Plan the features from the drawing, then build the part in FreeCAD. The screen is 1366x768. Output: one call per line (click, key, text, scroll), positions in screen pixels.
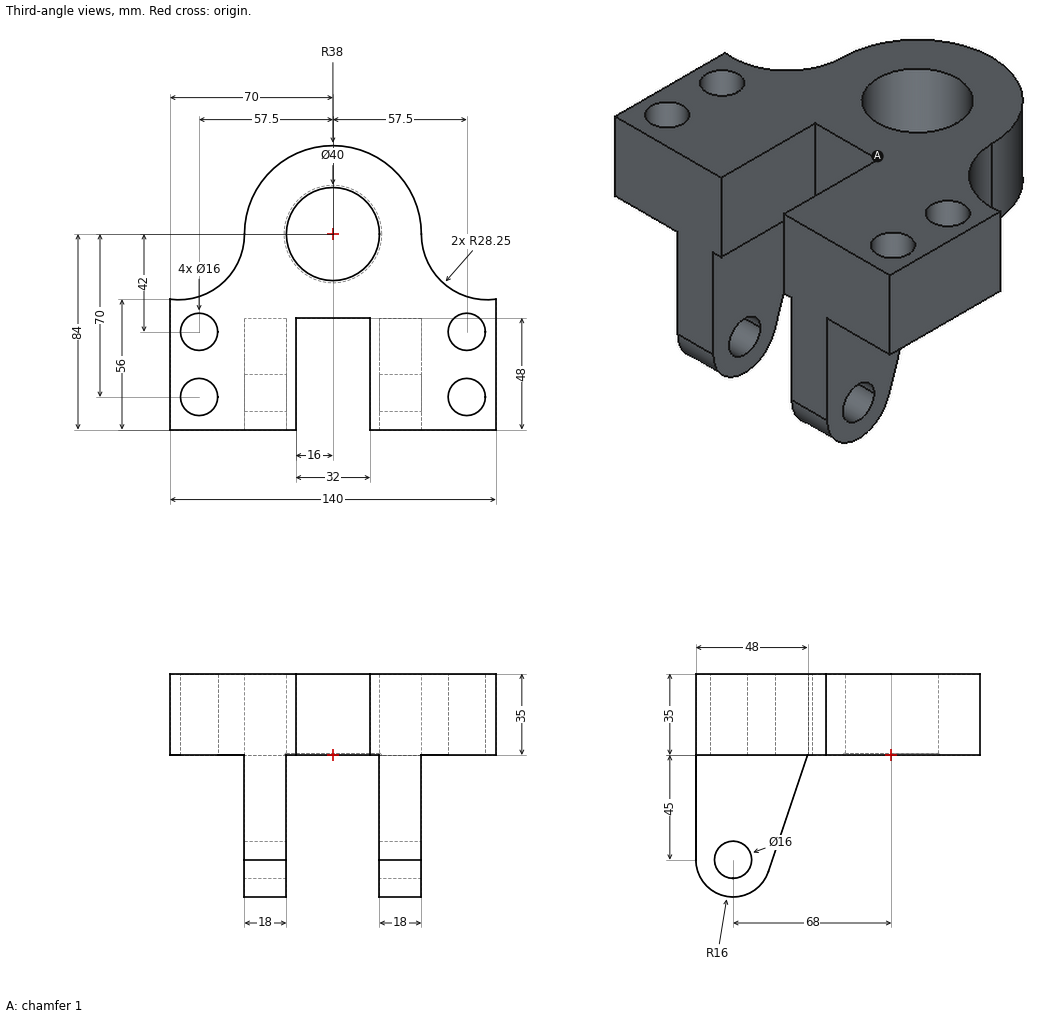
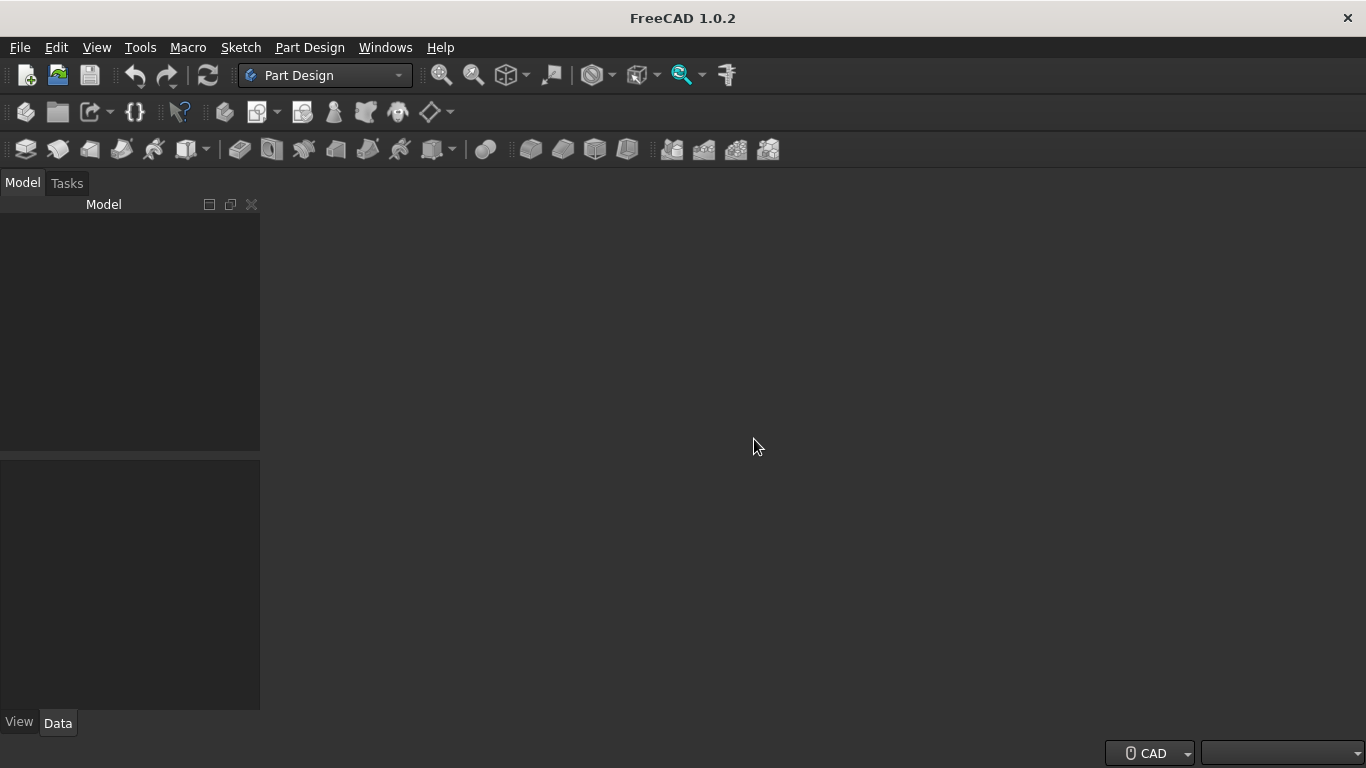
click(26, 76)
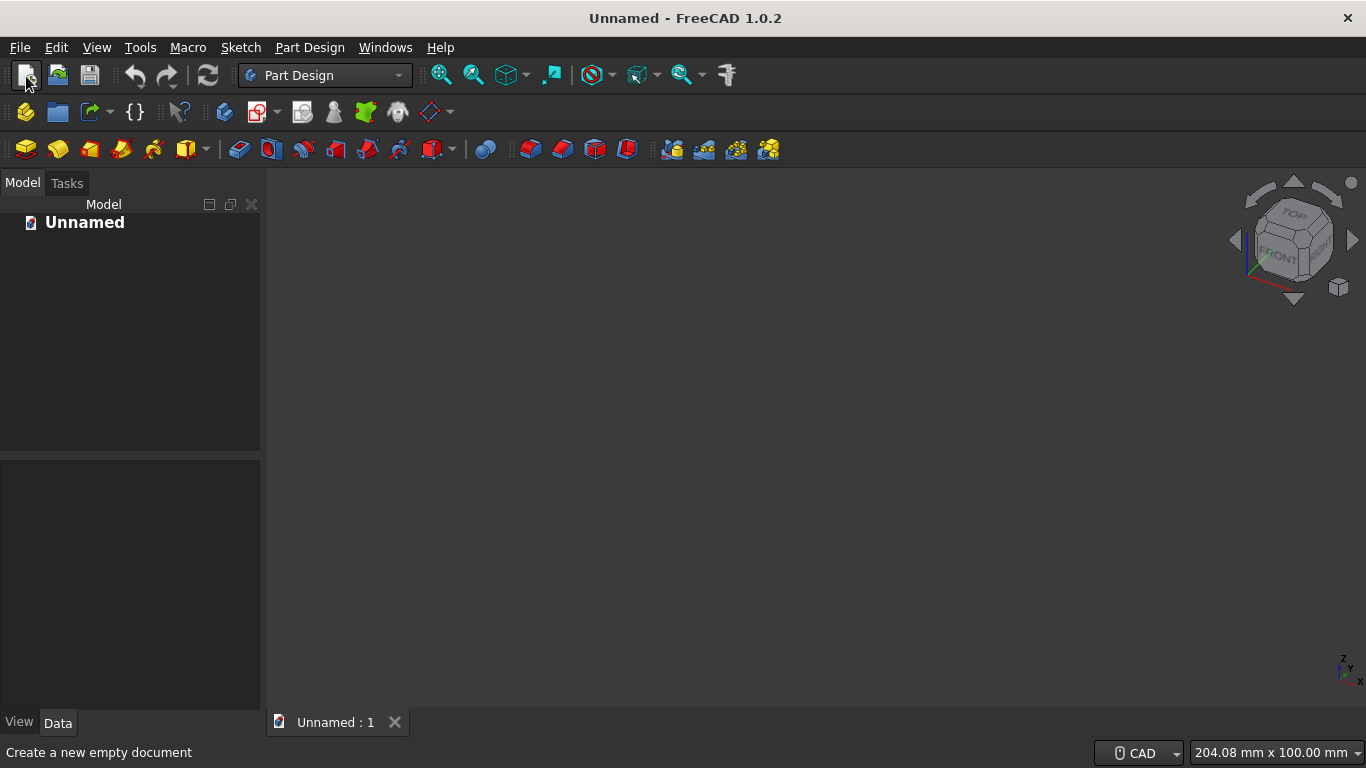
click(258, 112)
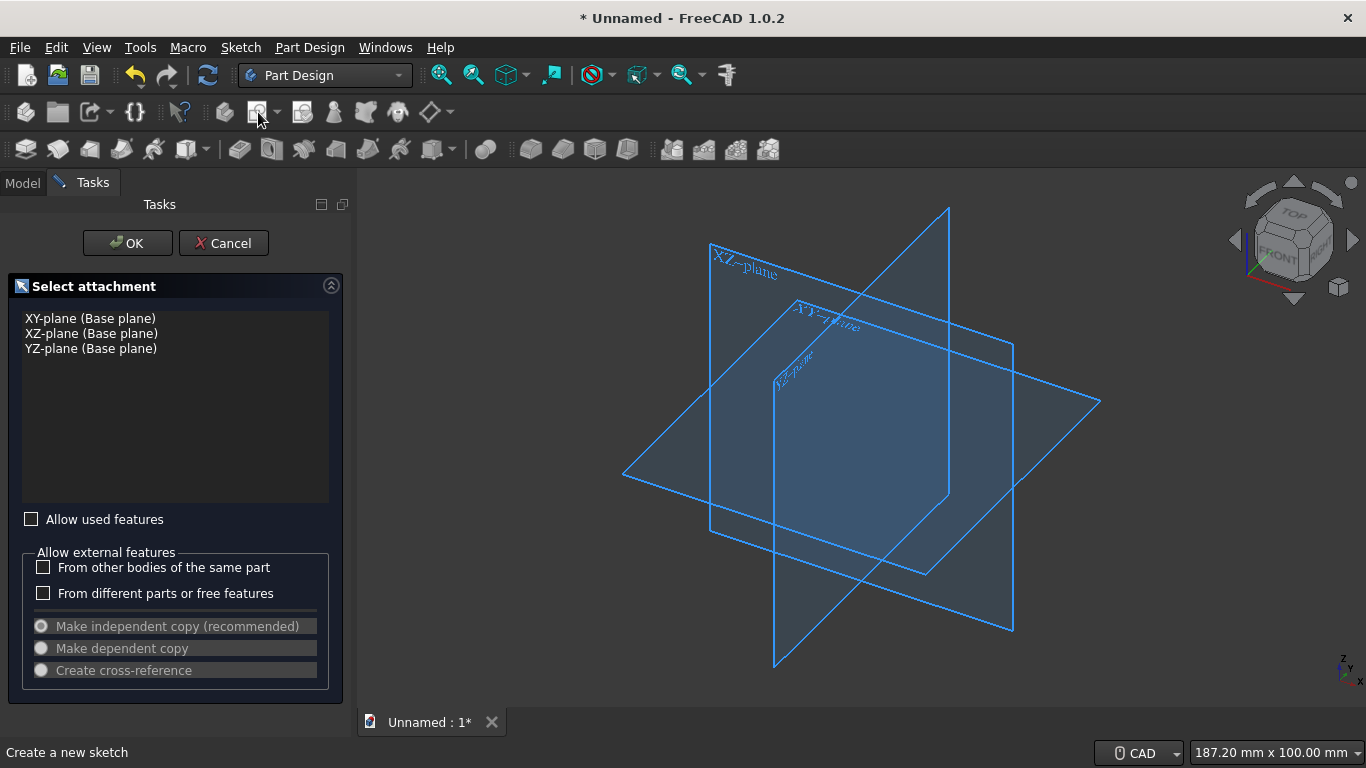
click(82, 318)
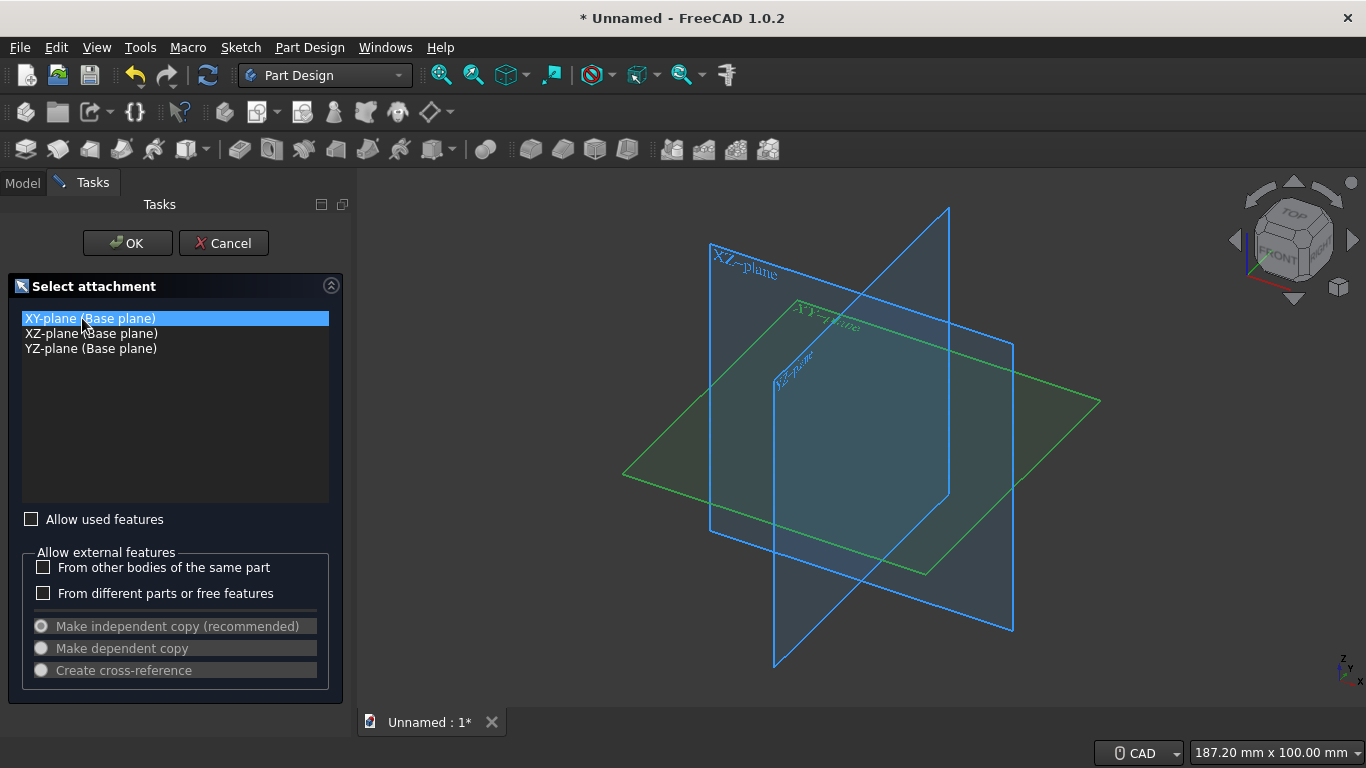
click(128, 243)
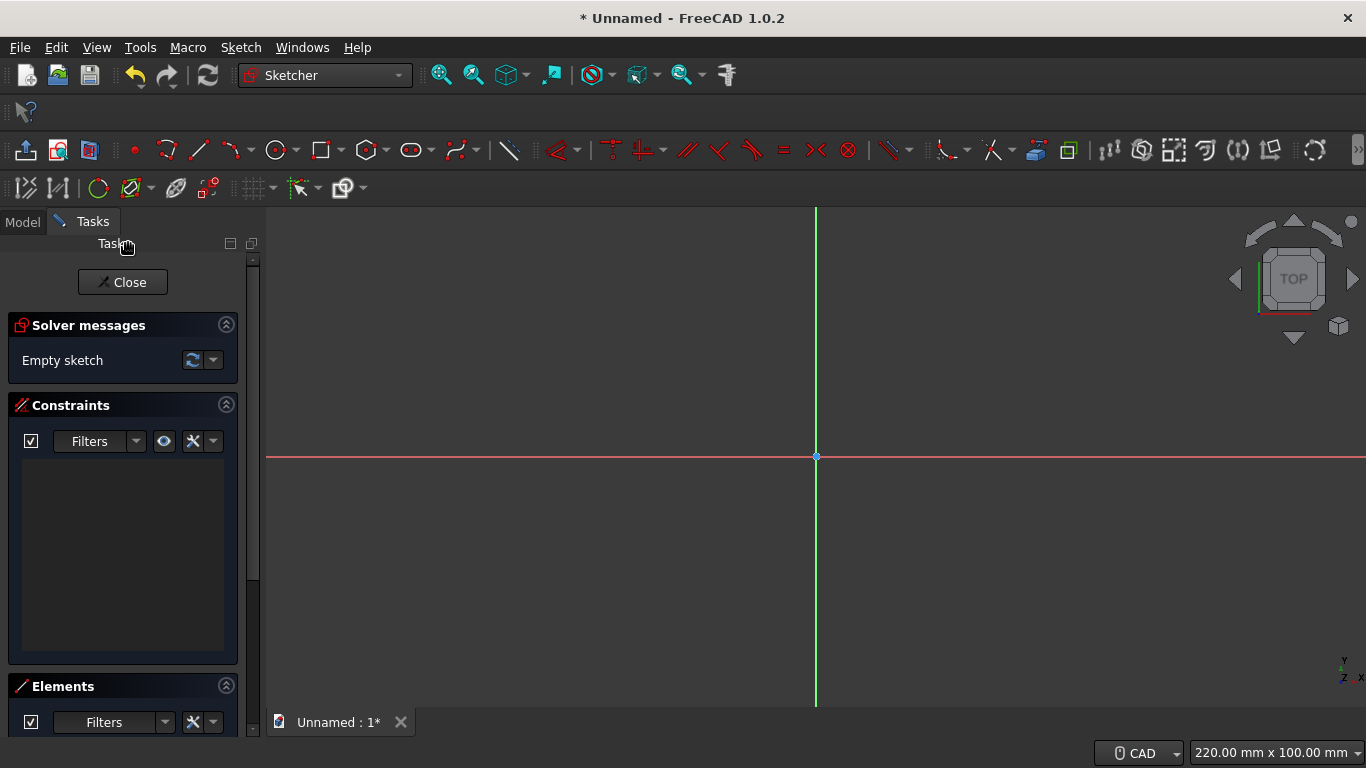
scroll(664, 317, down, 3)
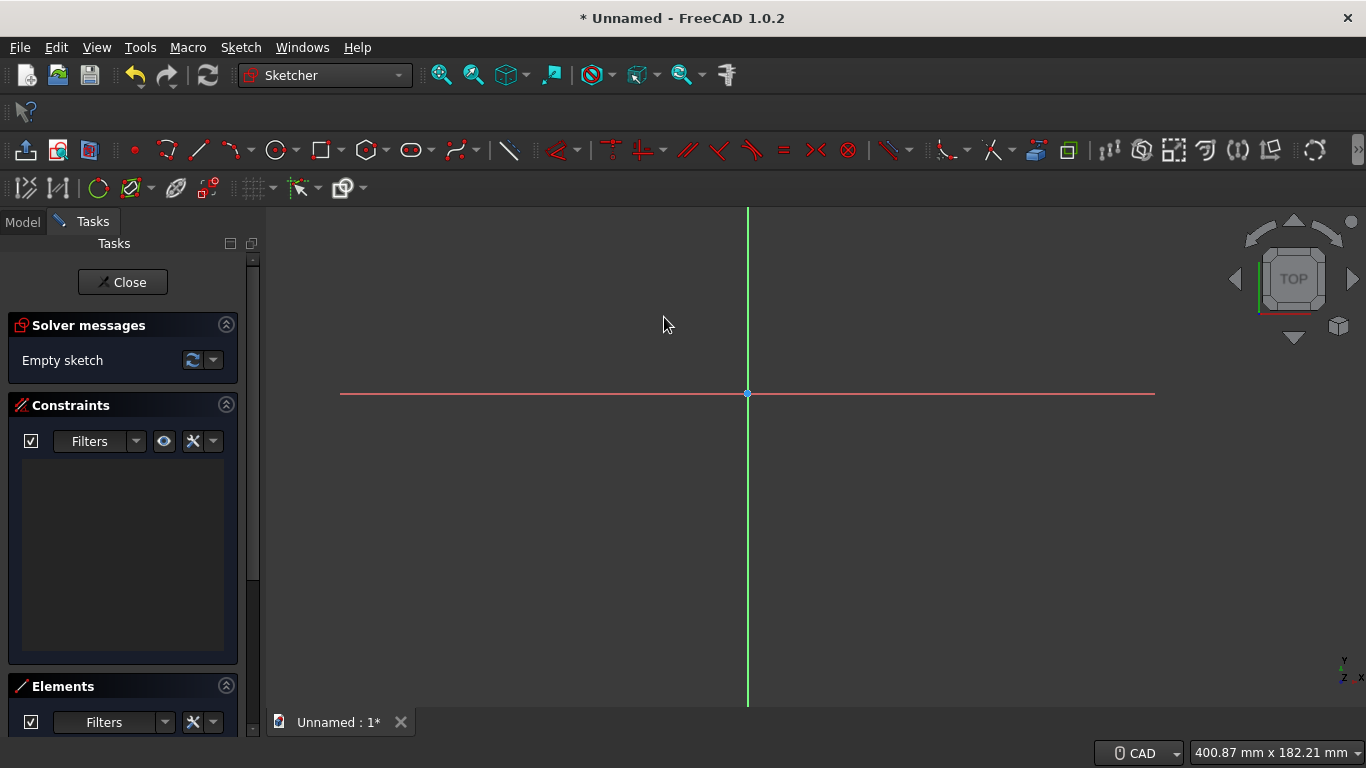
key(g)
key(m)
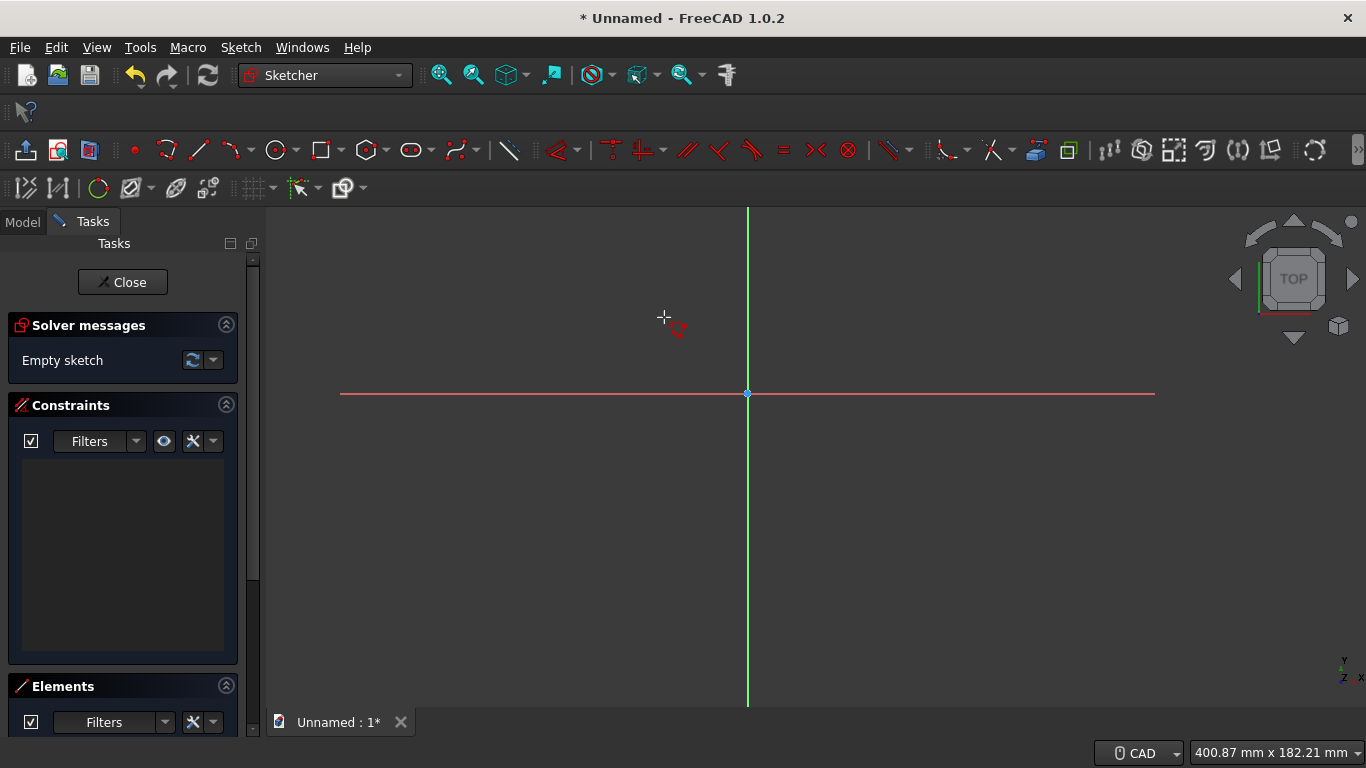
click(555, 471)
click(555, 624)
click(940, 624)
click(940, 471)
right_click(940, 471)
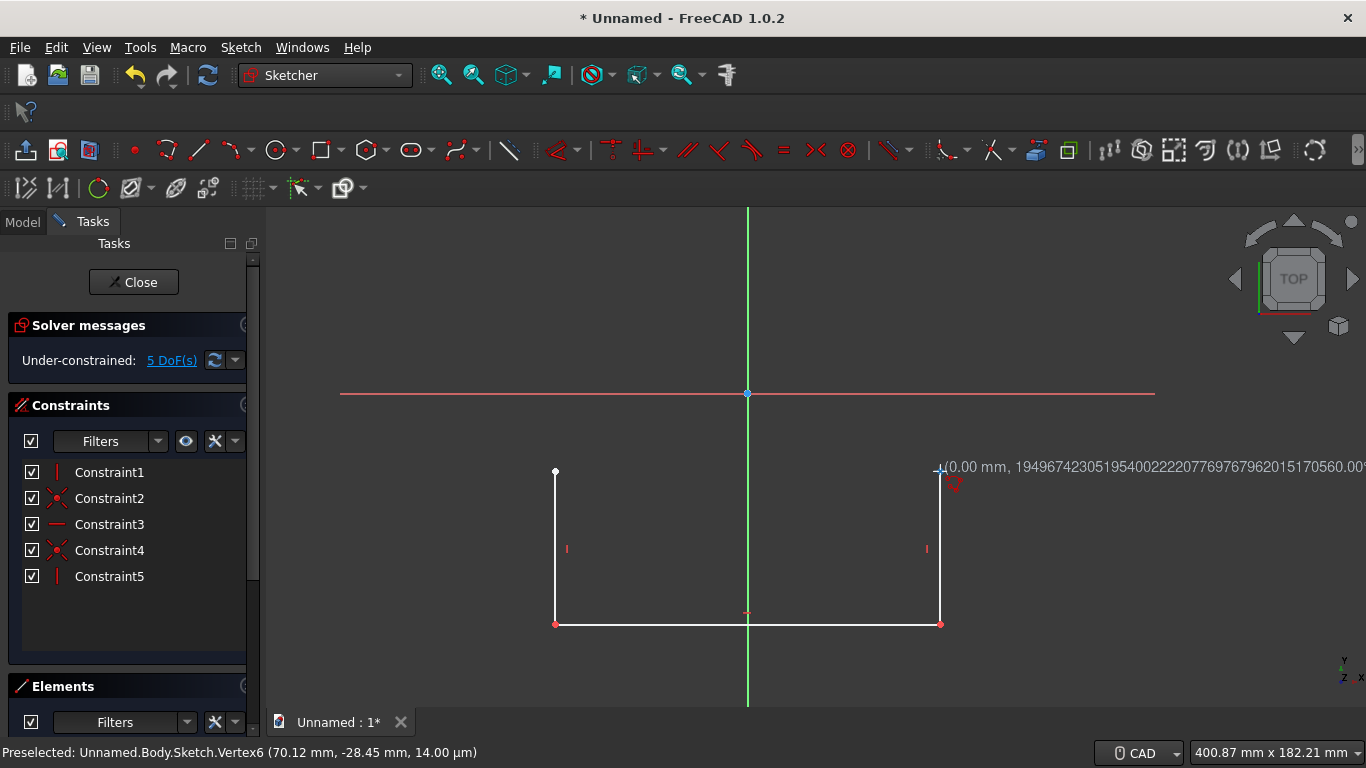
click(232, 150)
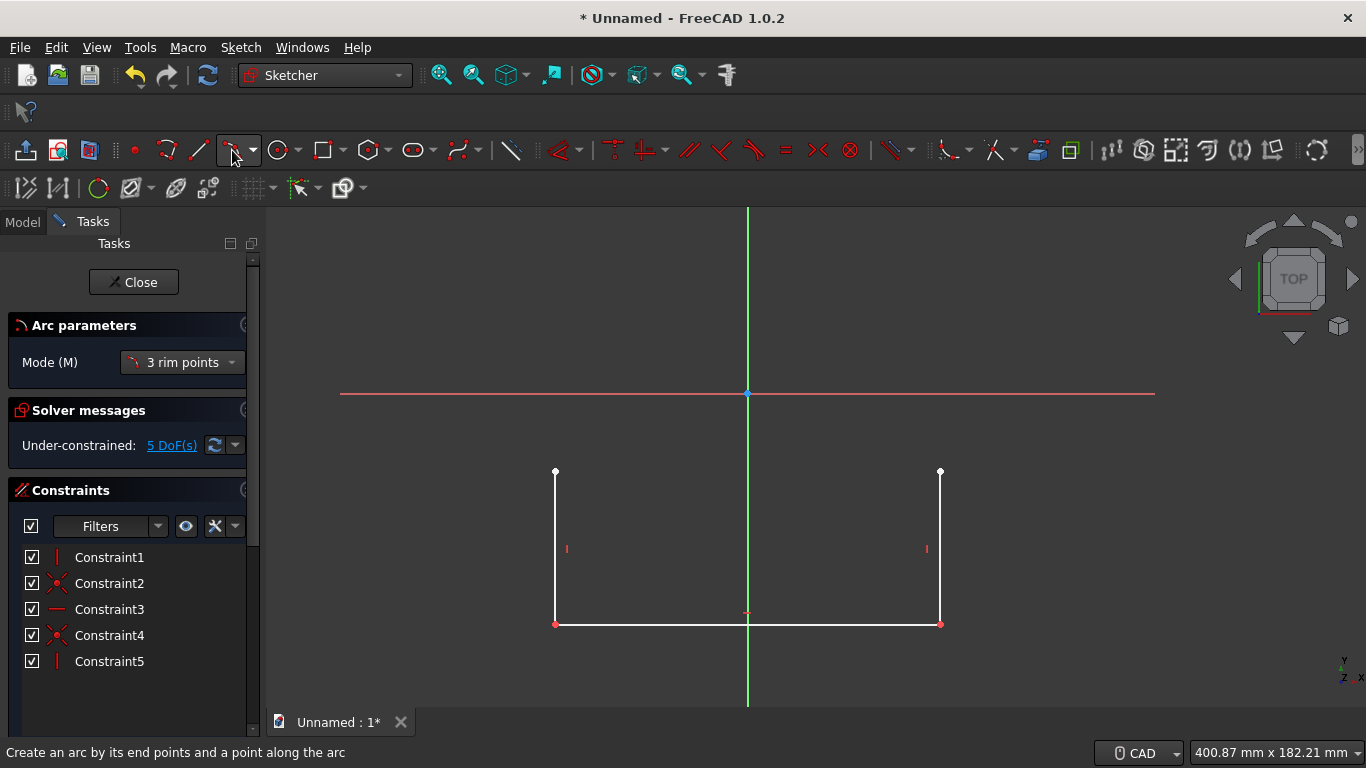
click(940, 472)
click(852, 394)
click(878, 452)